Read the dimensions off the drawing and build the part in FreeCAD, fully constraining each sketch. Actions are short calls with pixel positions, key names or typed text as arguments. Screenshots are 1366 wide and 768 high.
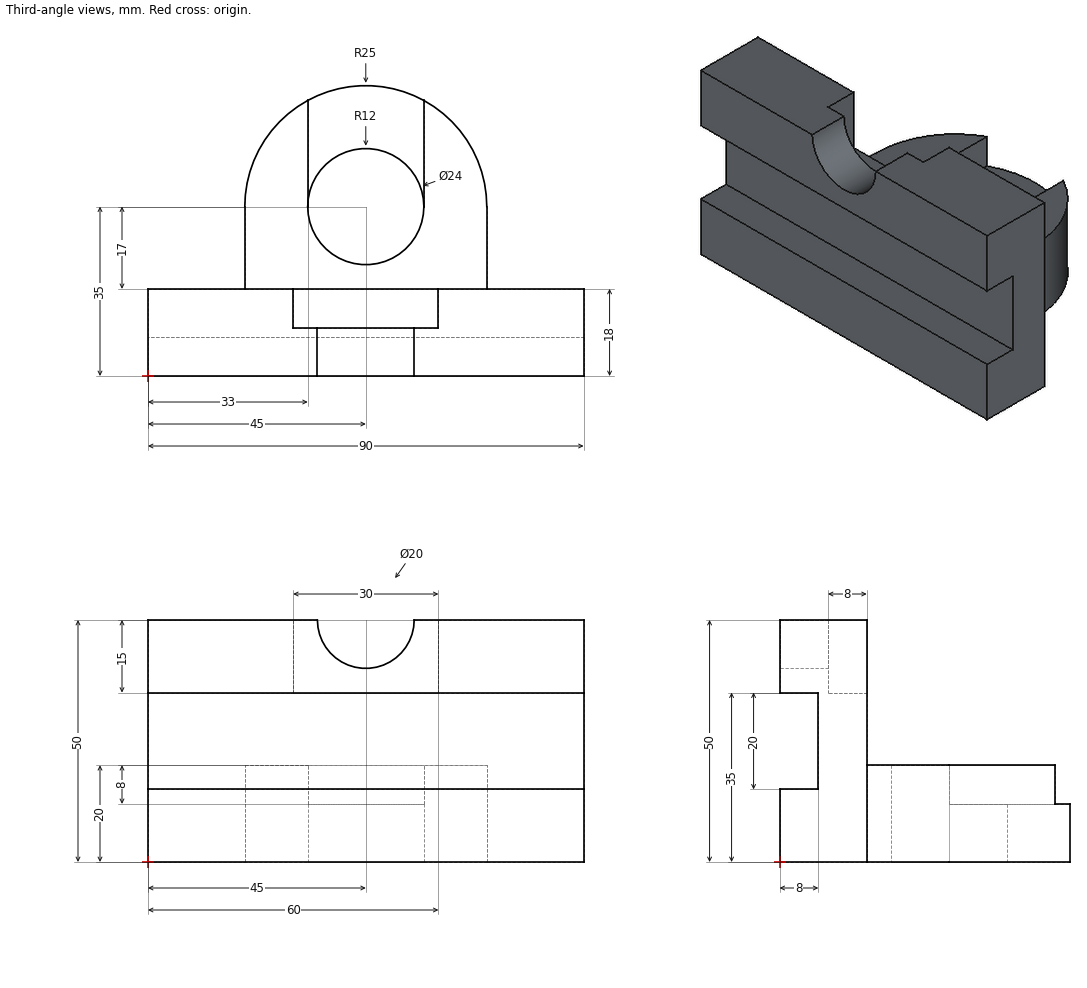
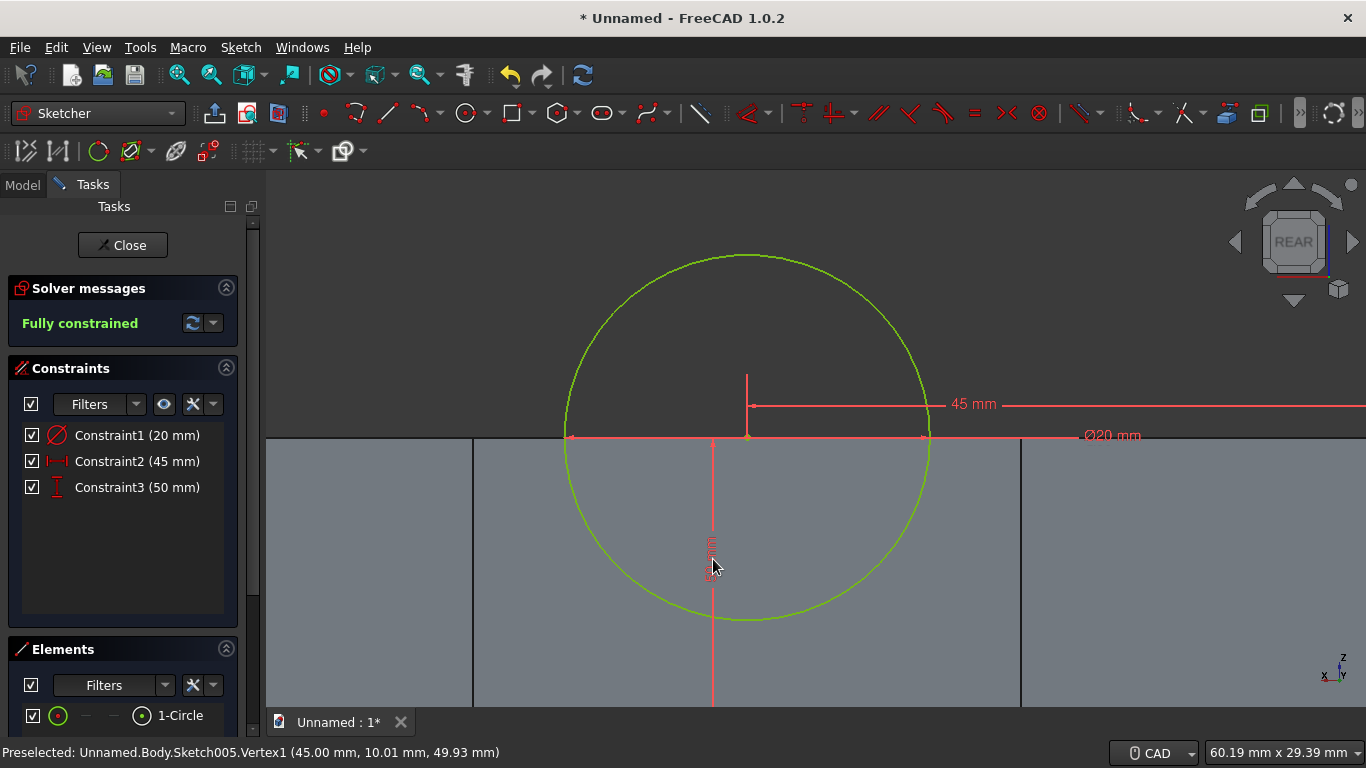
click(123, 245)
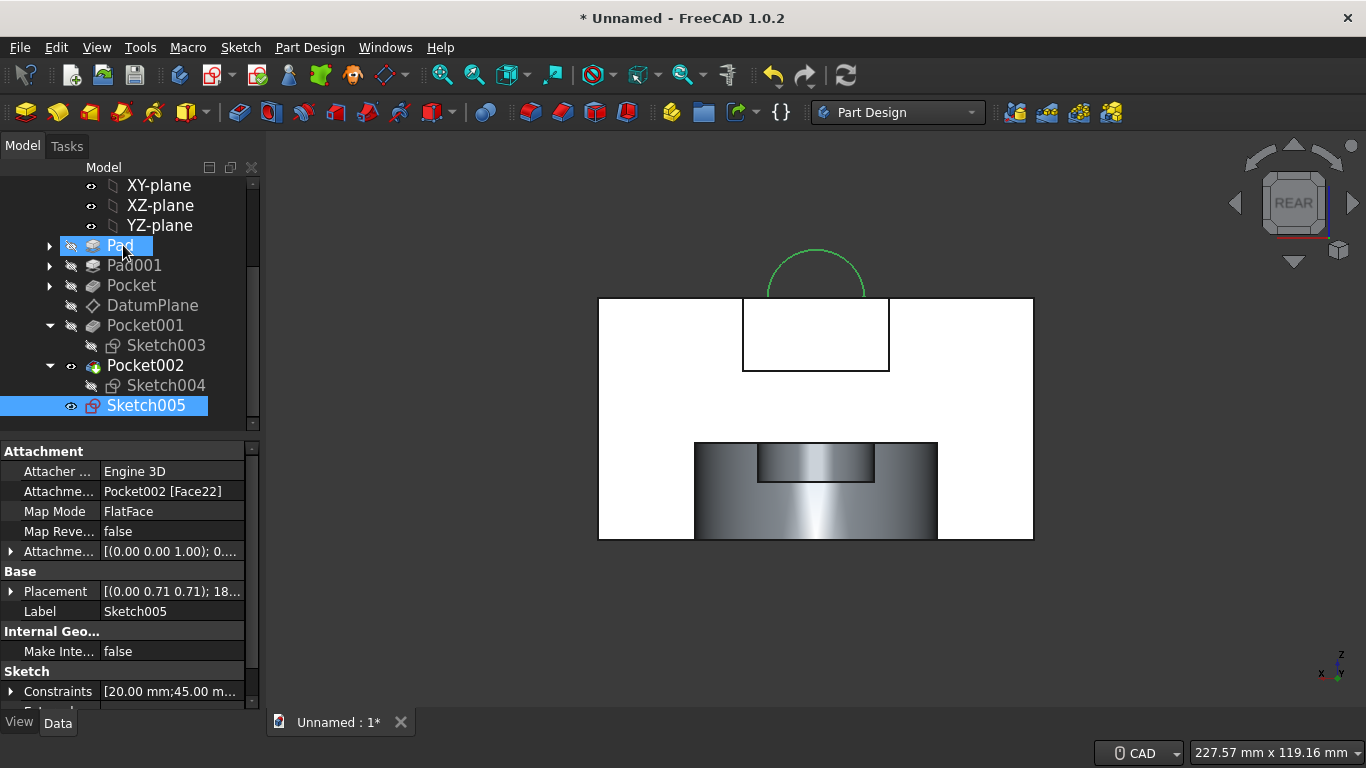
click(240, 112)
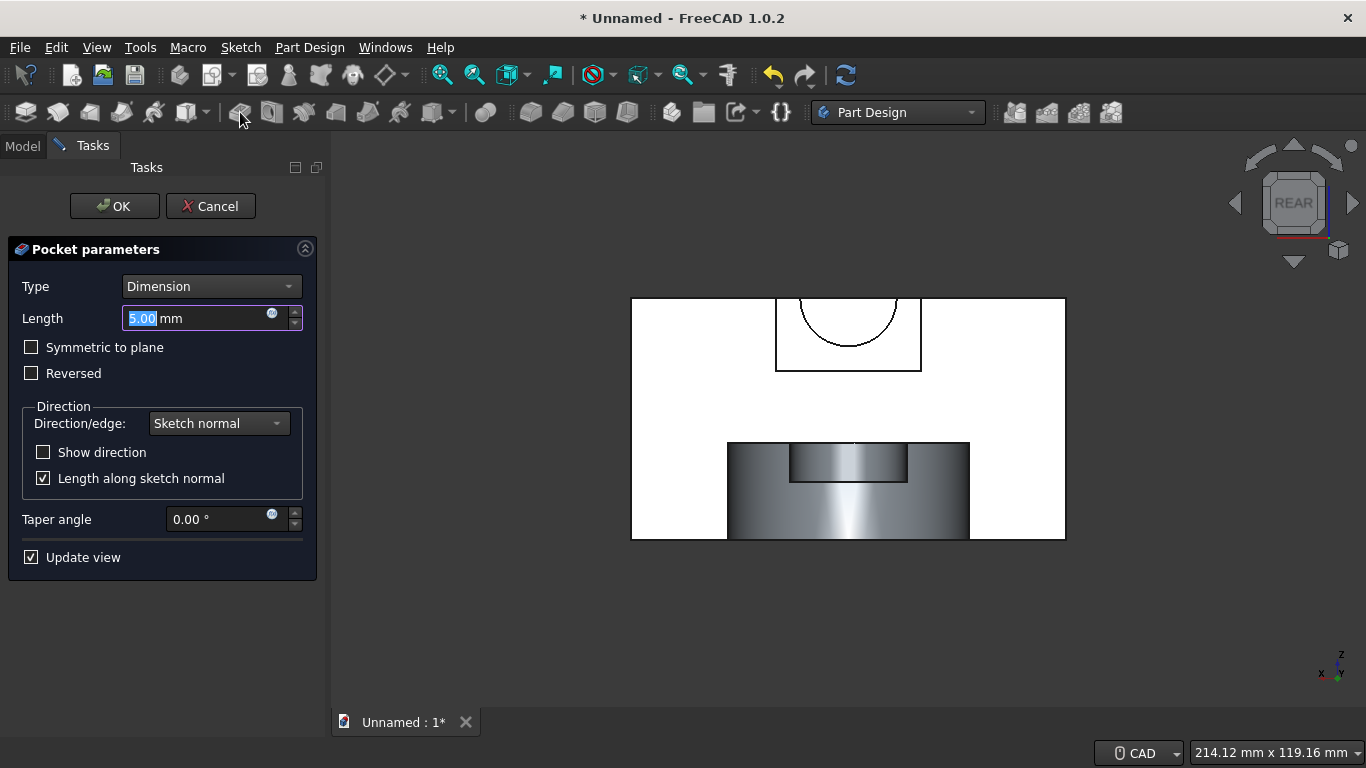
click(212, 286)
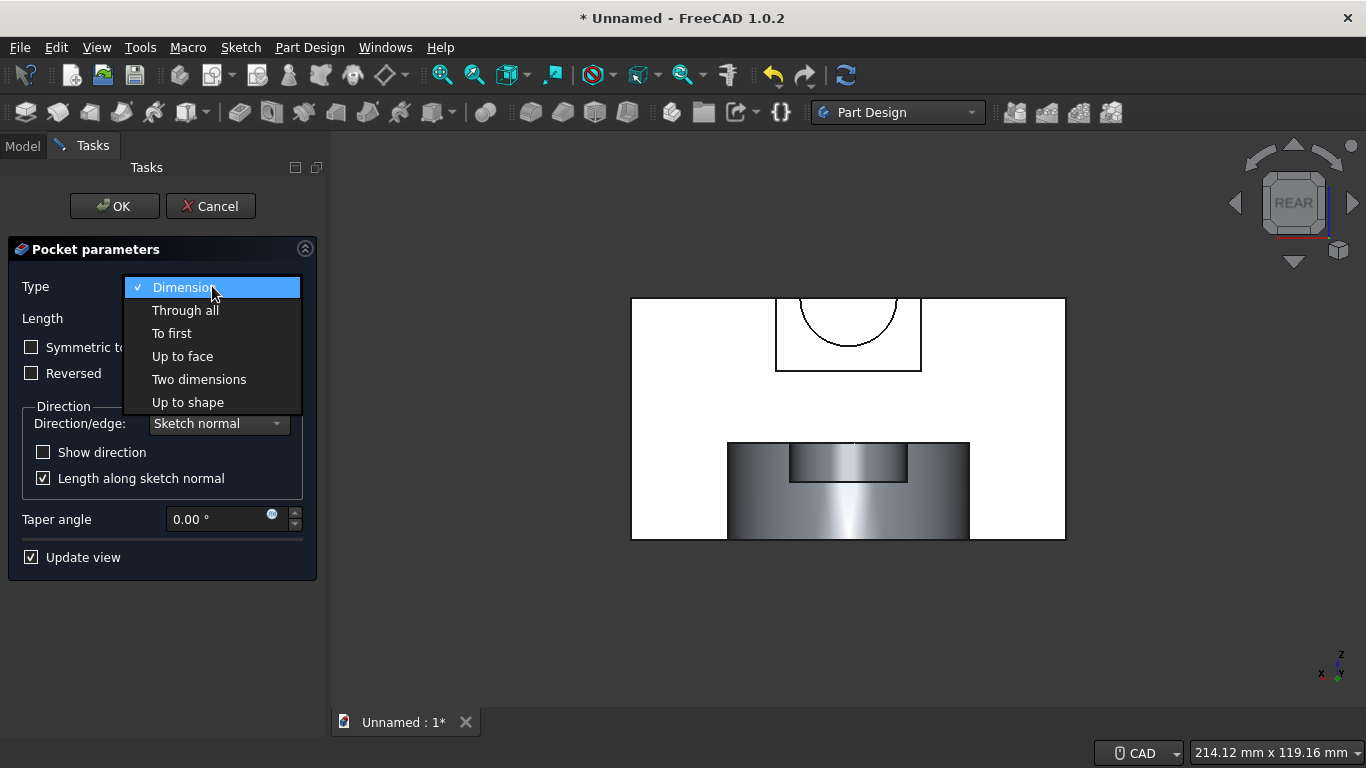
click(212, 310)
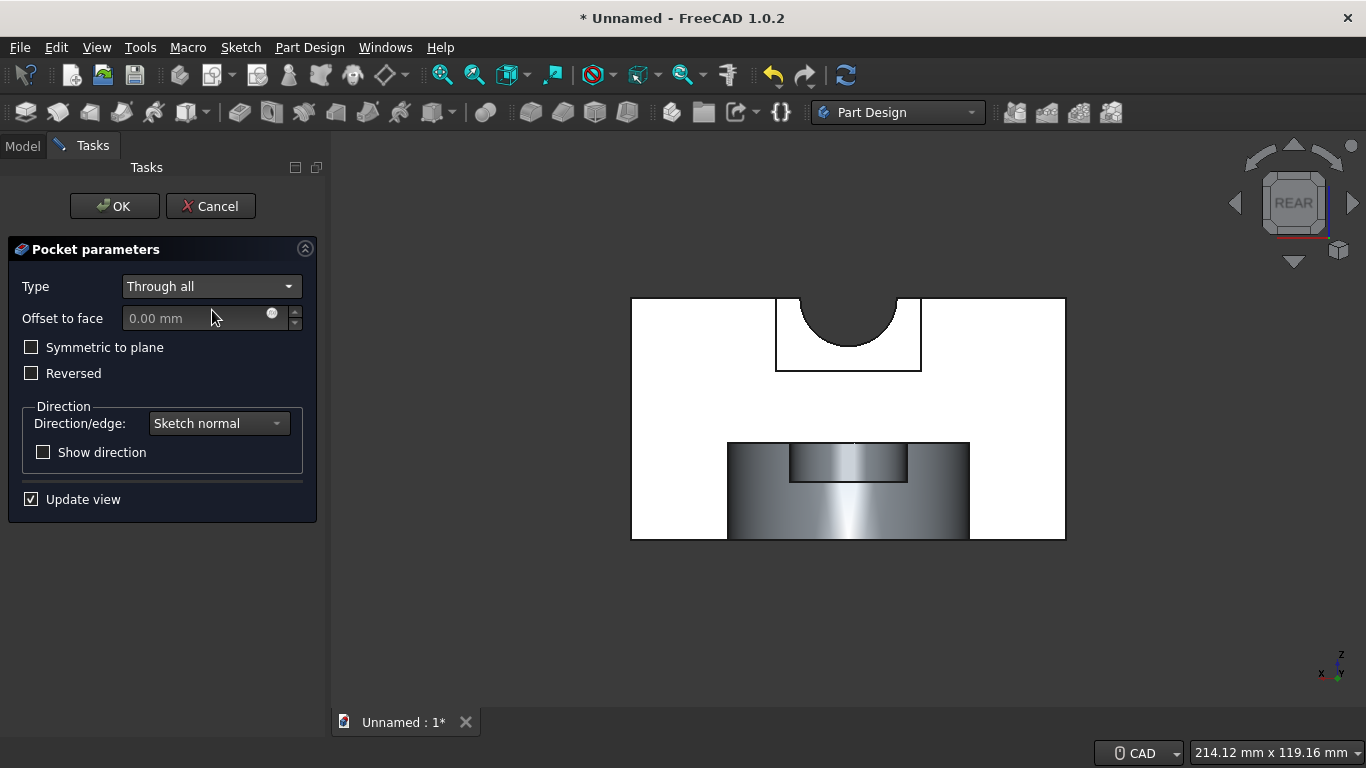
click(115, 206)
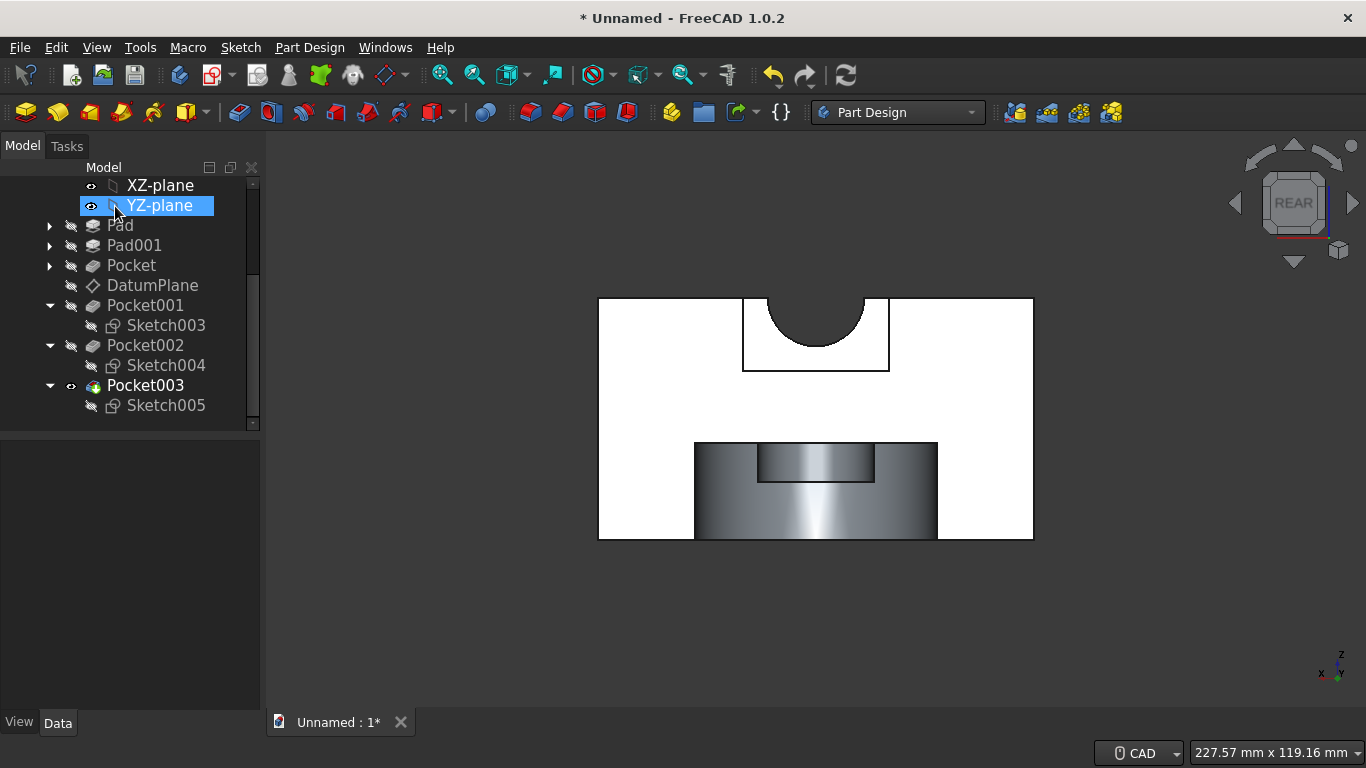
key(0)